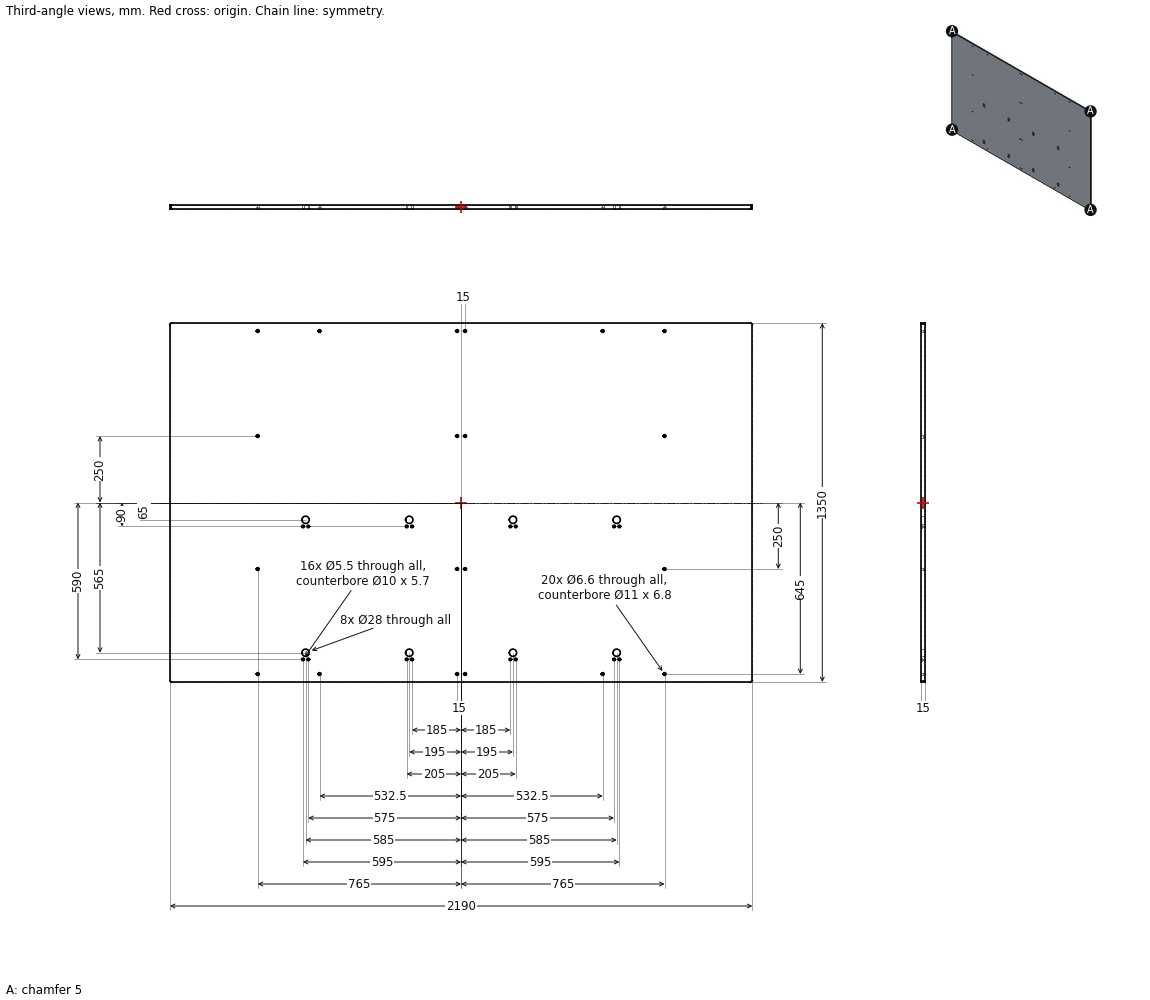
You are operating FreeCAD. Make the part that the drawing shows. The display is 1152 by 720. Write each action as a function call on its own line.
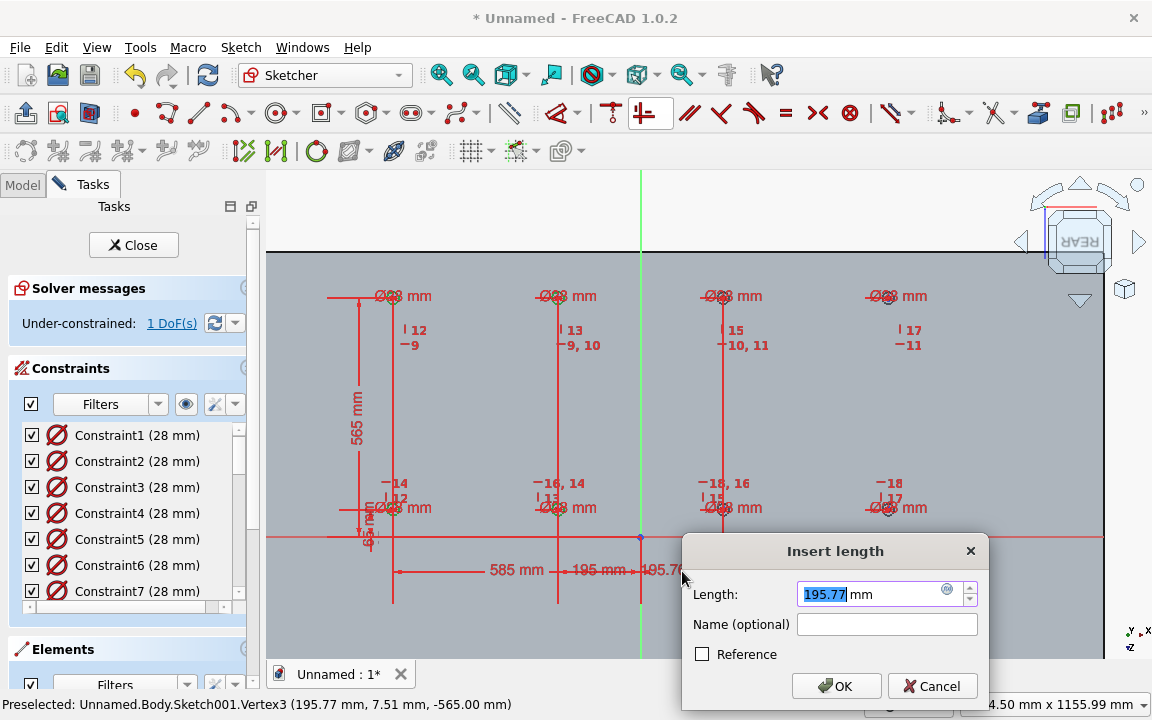
text(195)
key(Return)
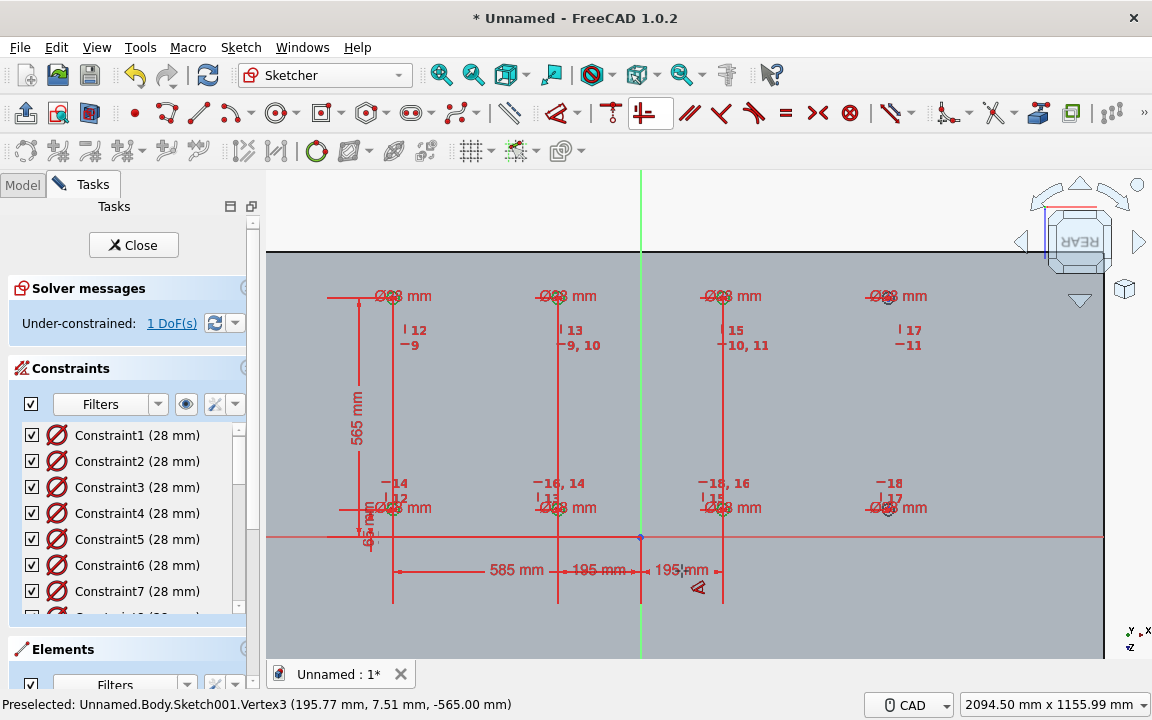
click(888, 298)
click(764, 571)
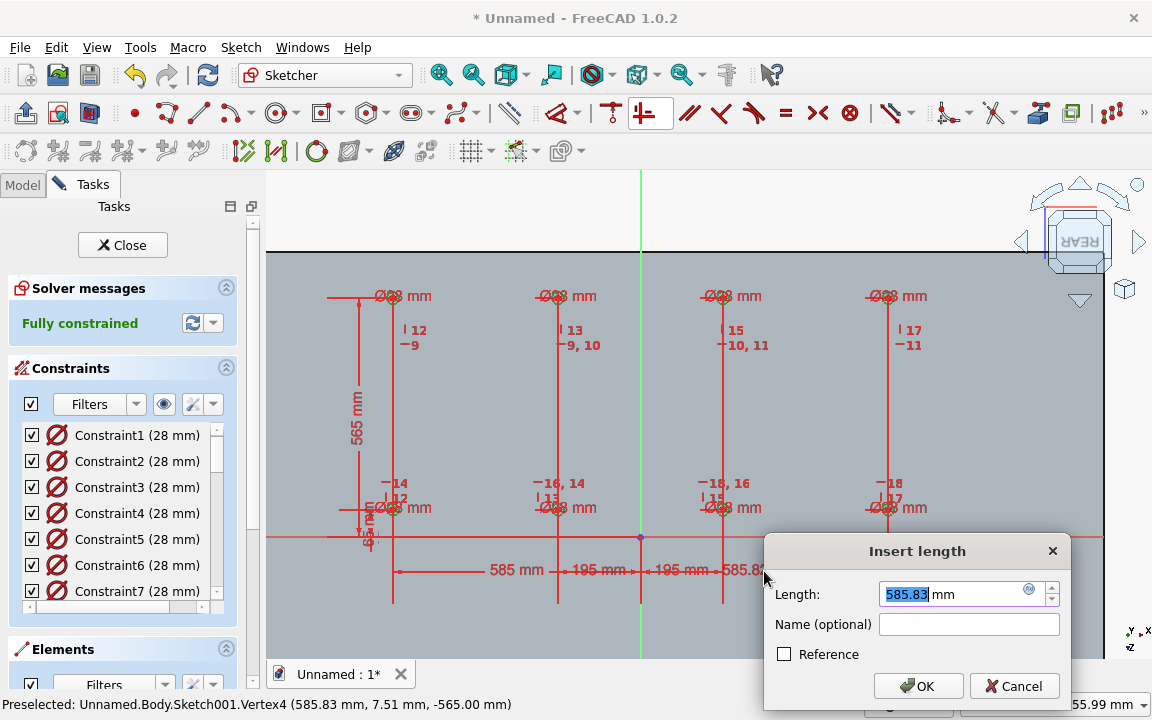
text(585)
key(Return)
key(Escape)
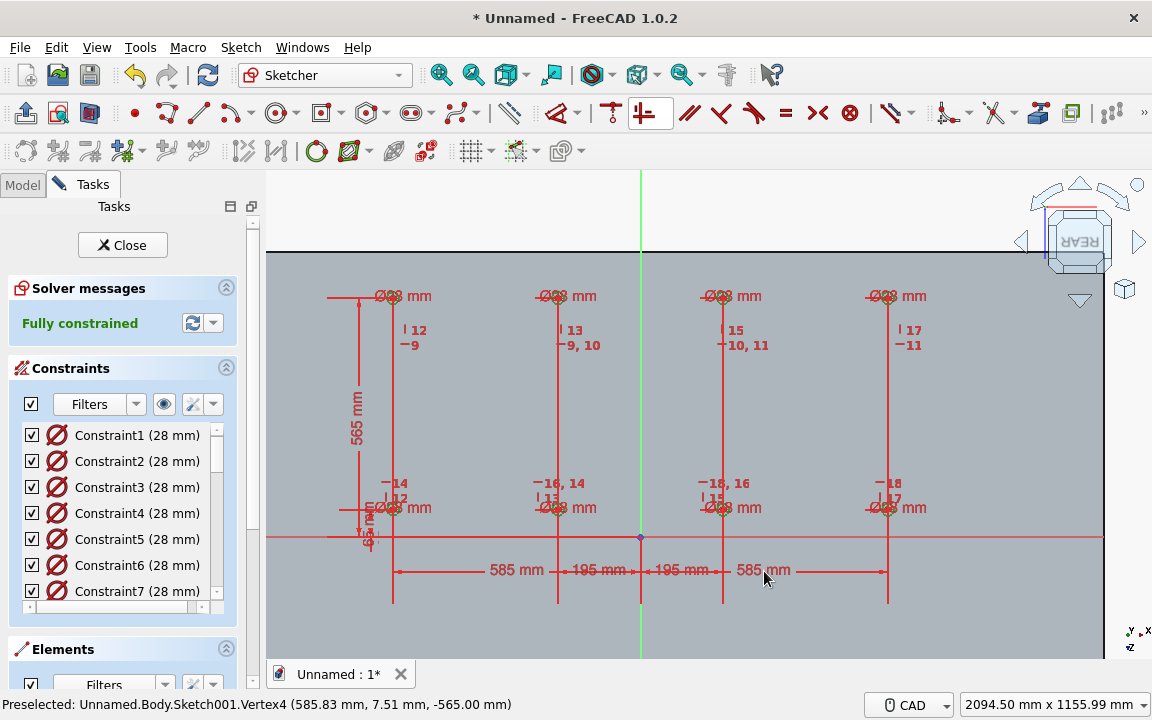
click(123, 245)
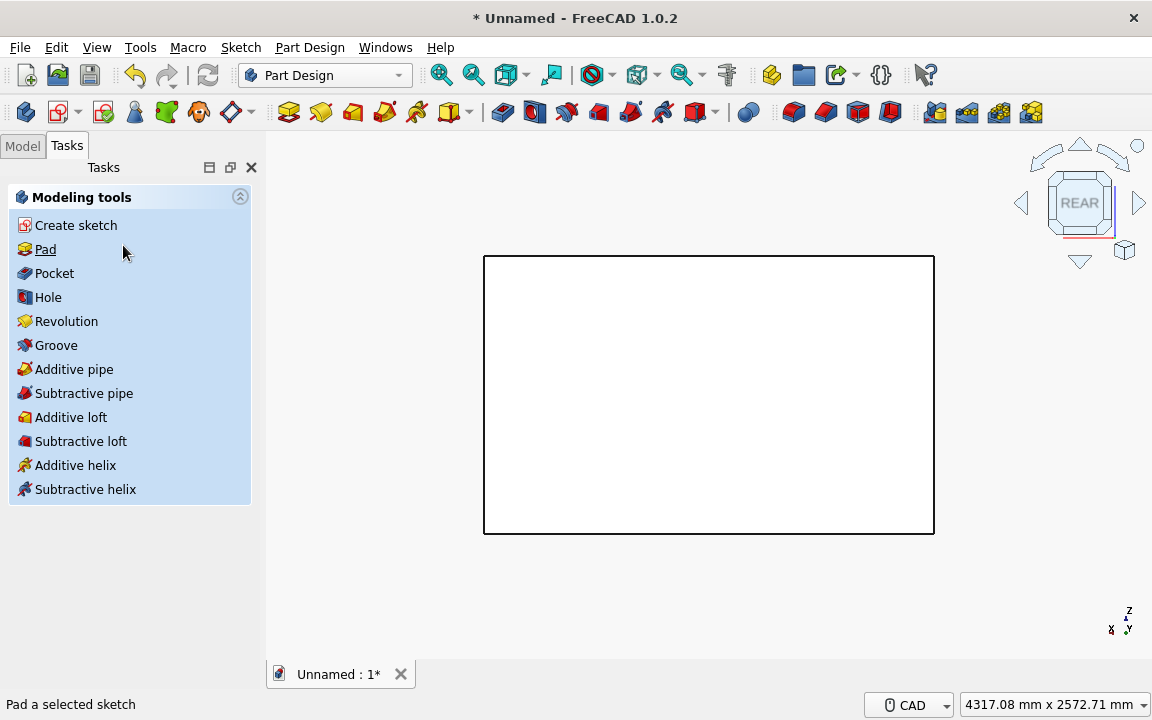
click(536, 112)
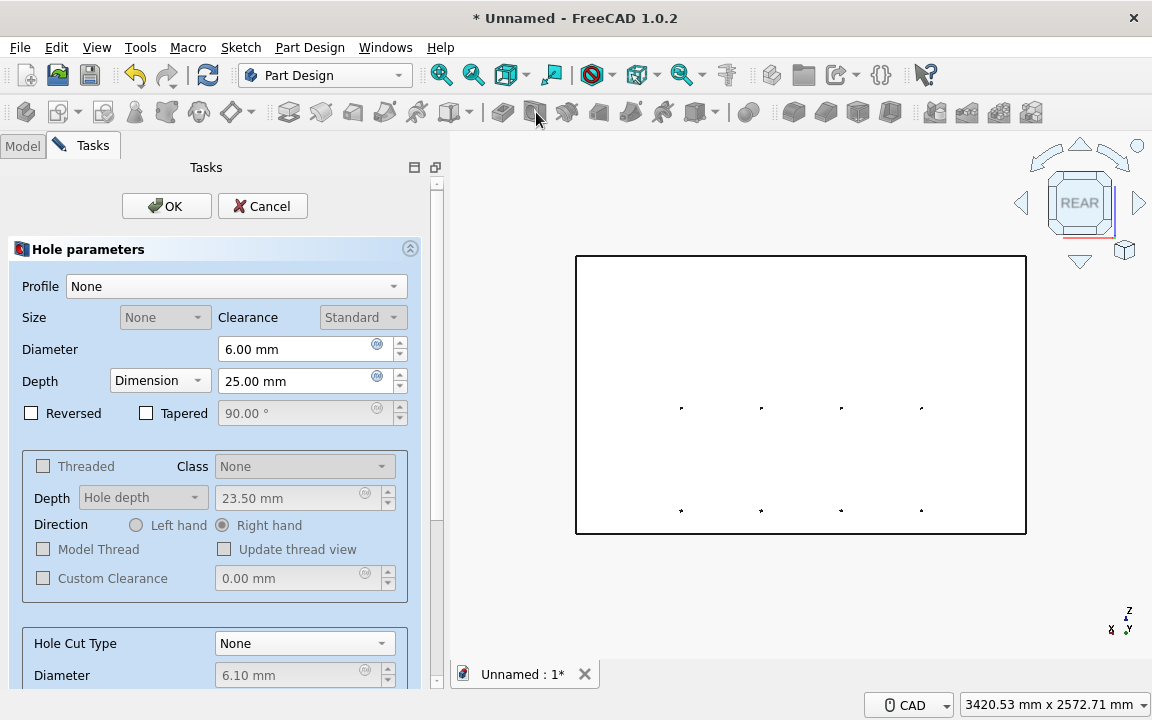
triple_click(305, 349)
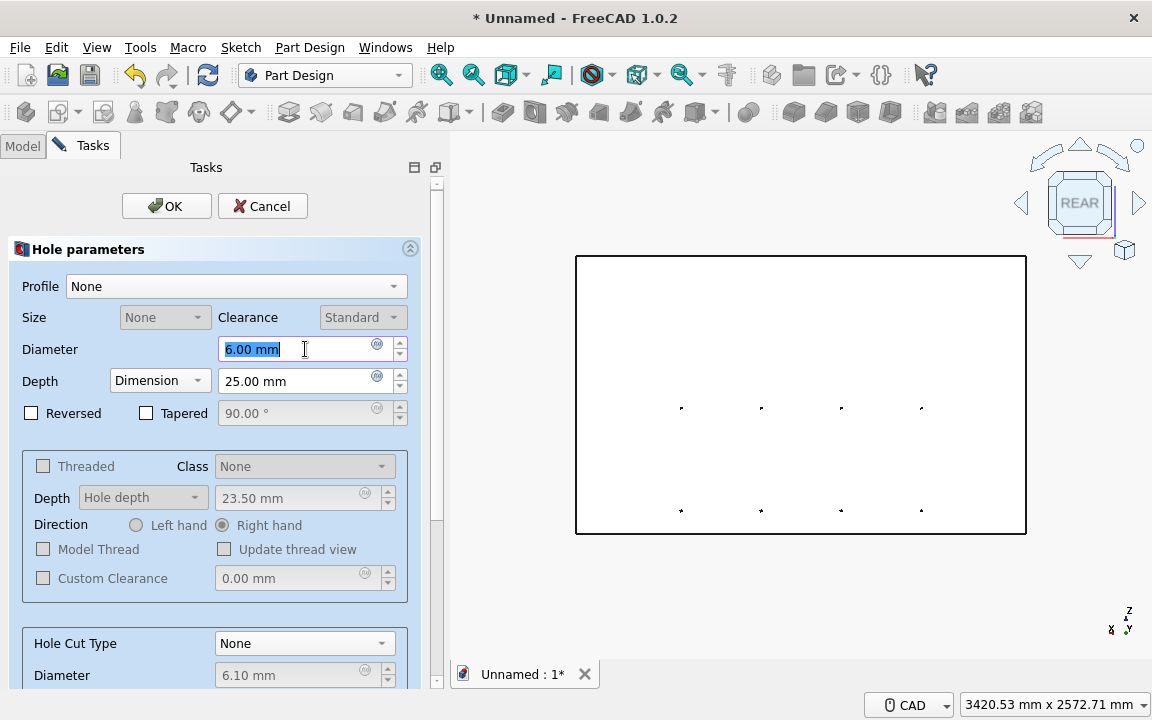
text(28)
key(Tab)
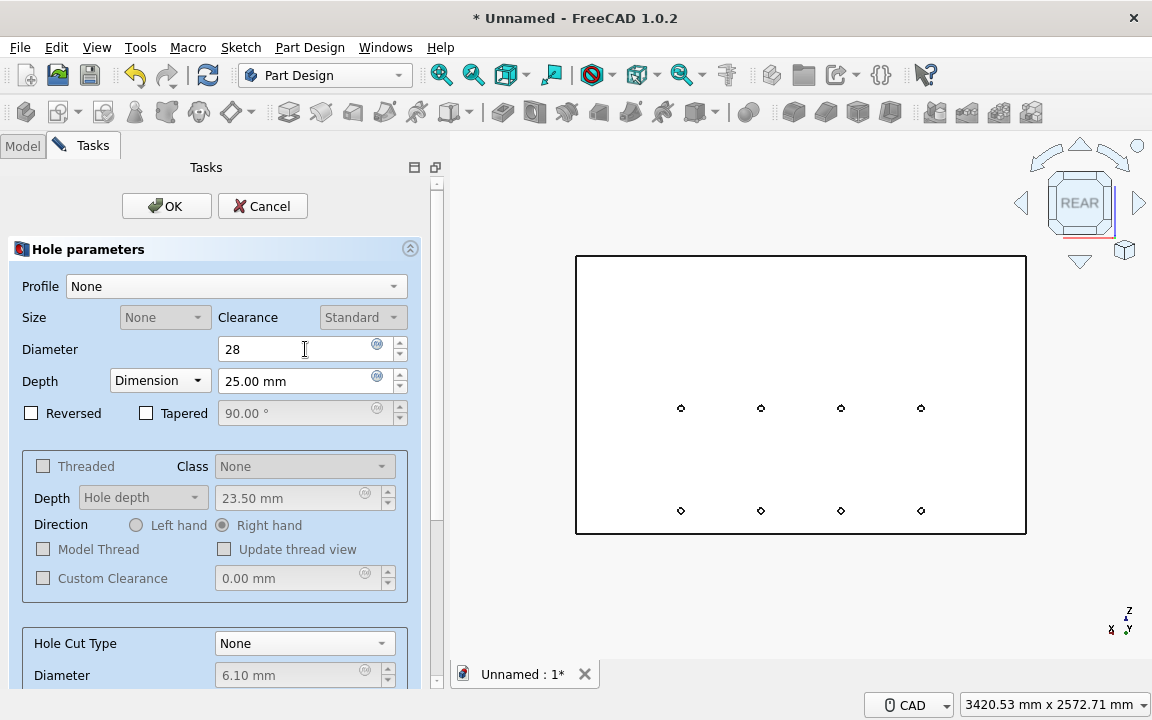
click(161, 380)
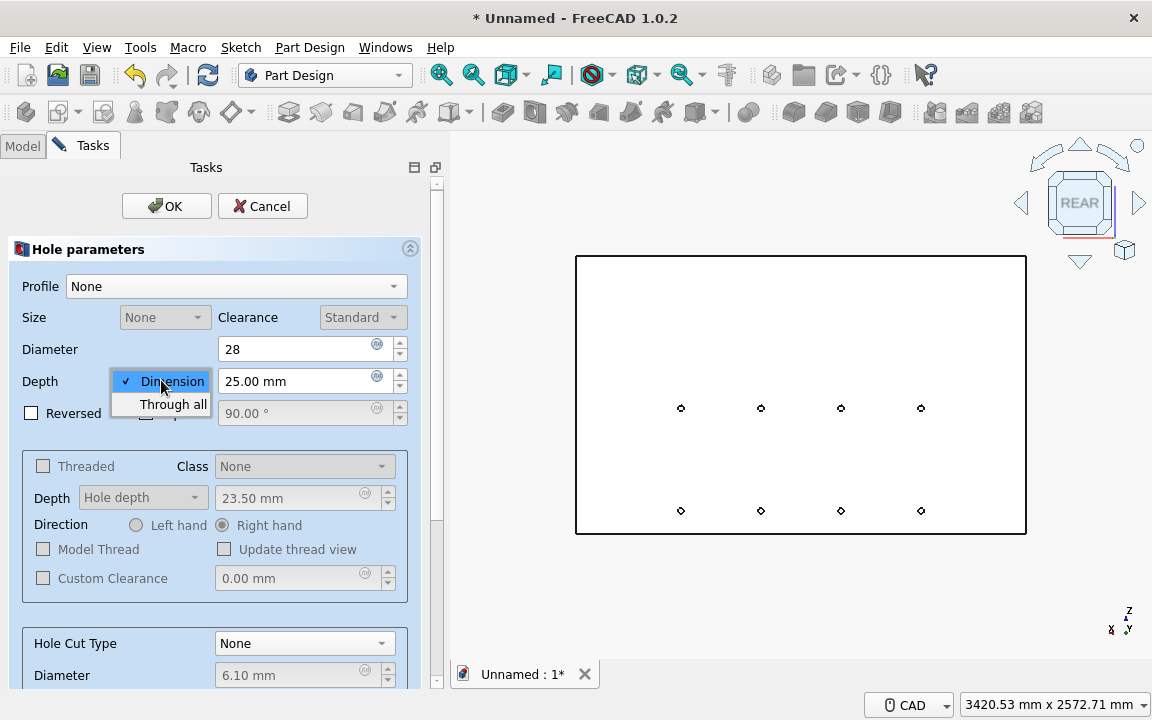
click(160, 404)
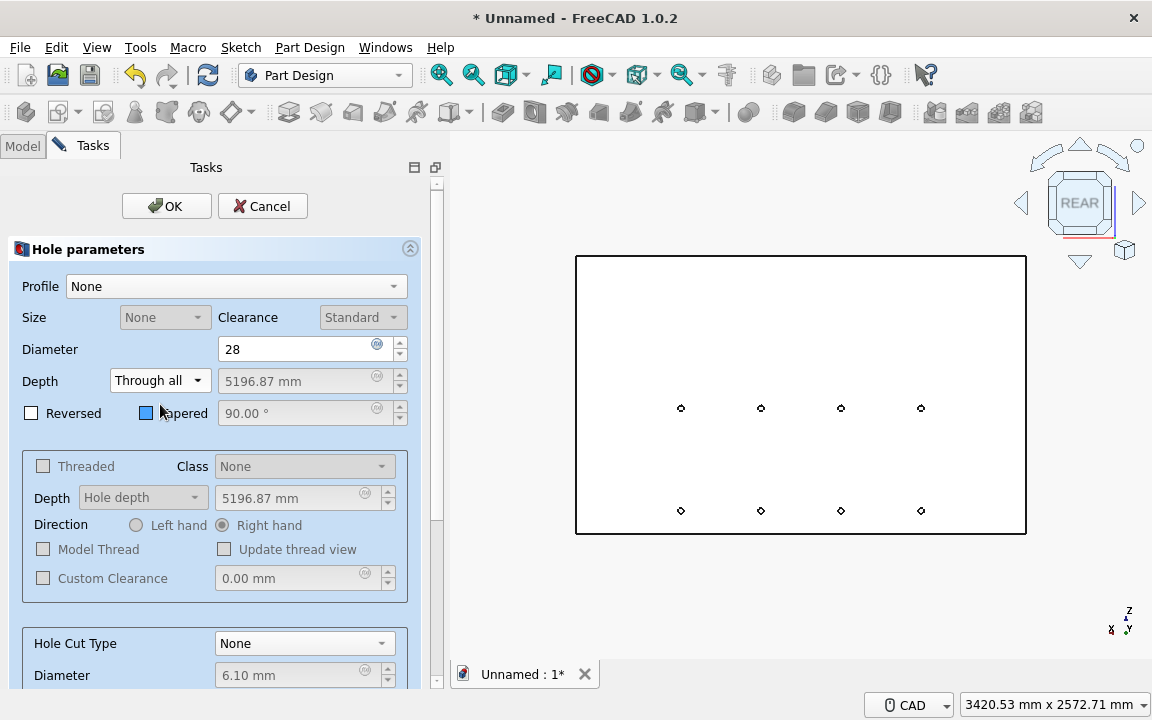
click(167, 206)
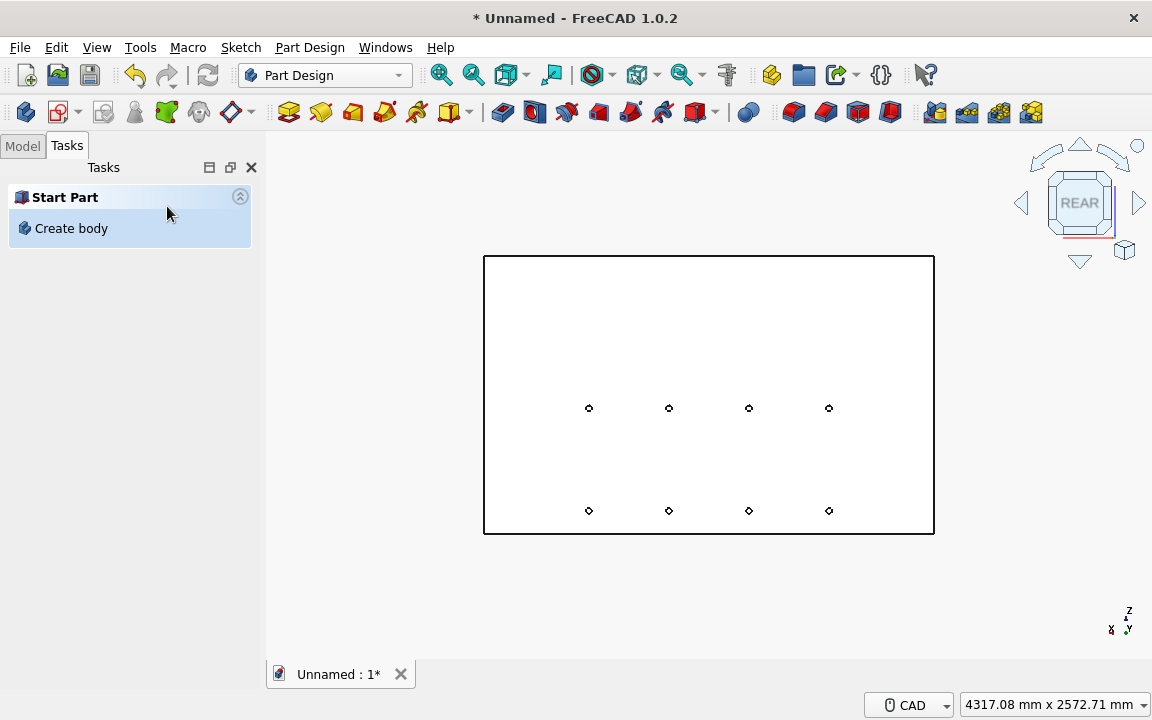
key(0)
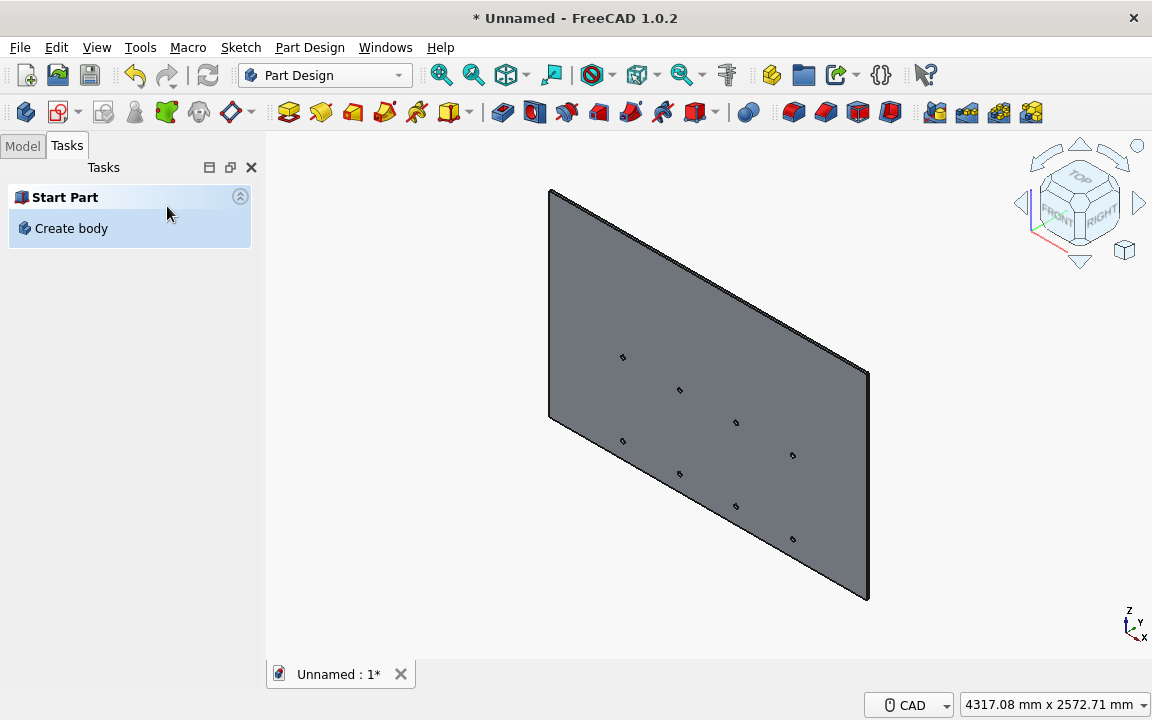
click(708, 362)